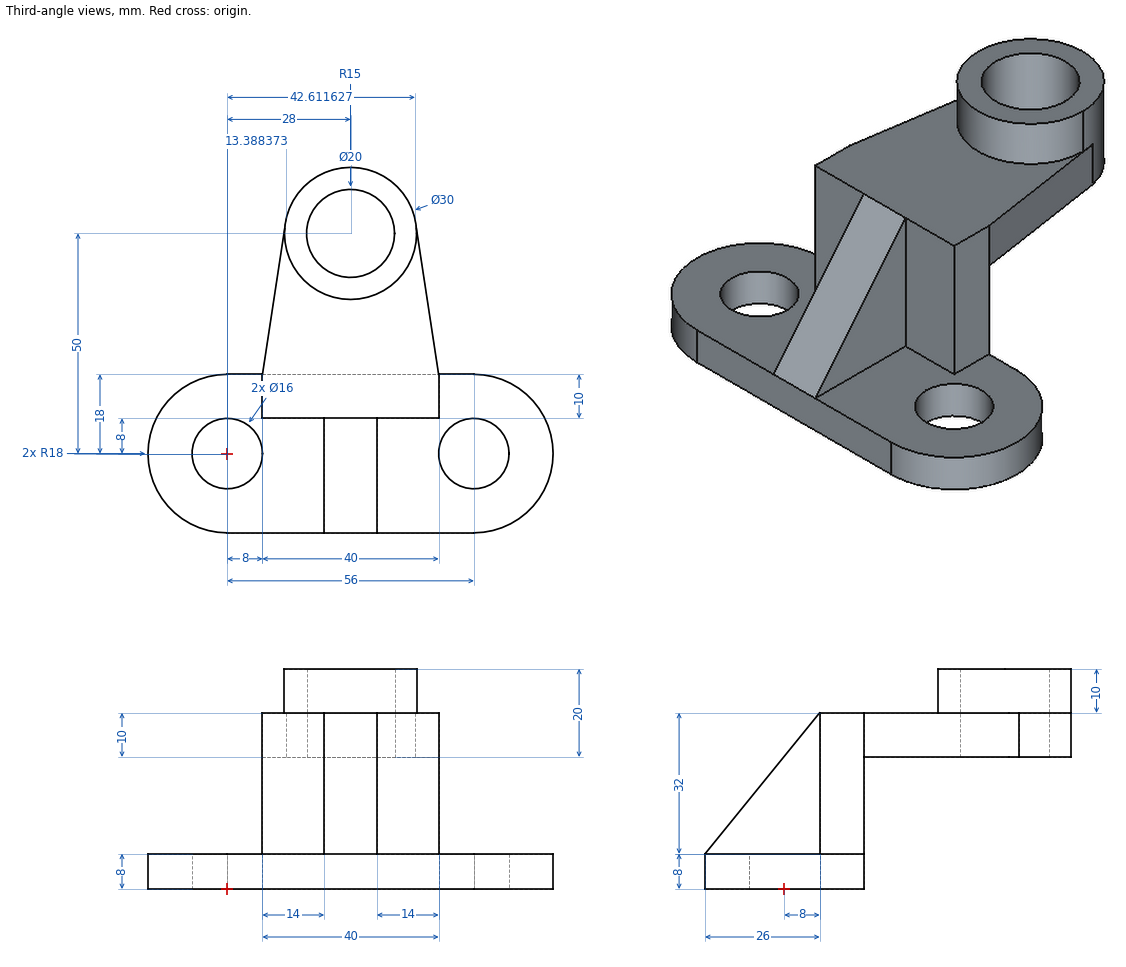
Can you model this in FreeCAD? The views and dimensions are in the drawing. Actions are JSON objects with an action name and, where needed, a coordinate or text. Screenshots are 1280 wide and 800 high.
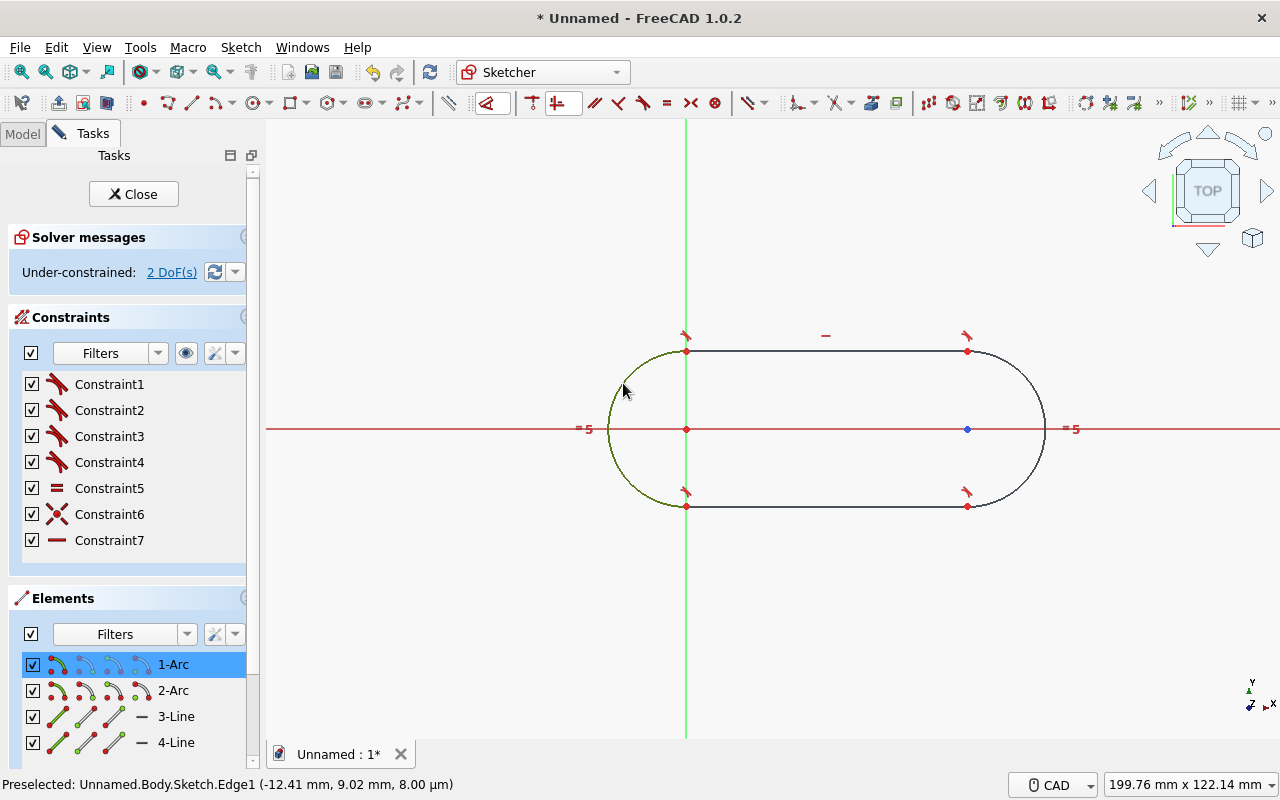
{"action": "key", "text": "k r"}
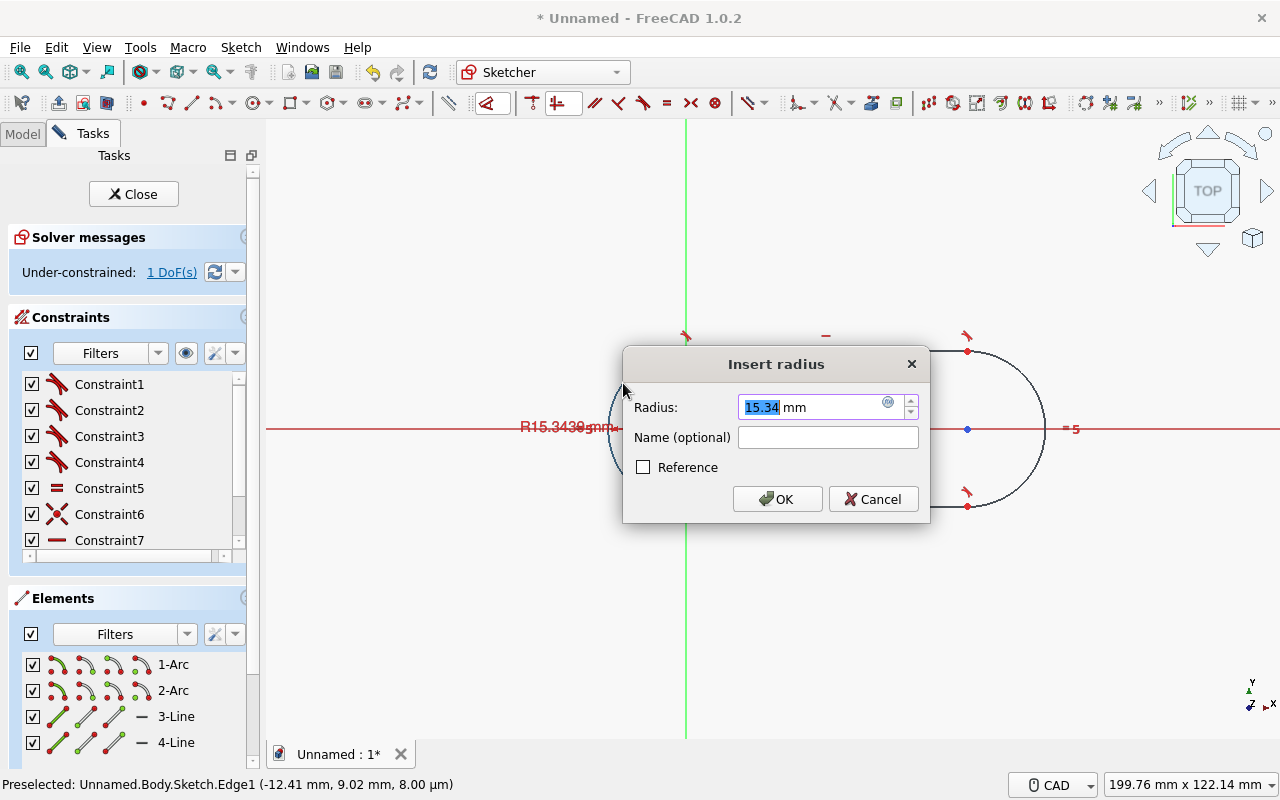
{"action": "type", "text": "18"}
{"action": "key", "text": "Return"}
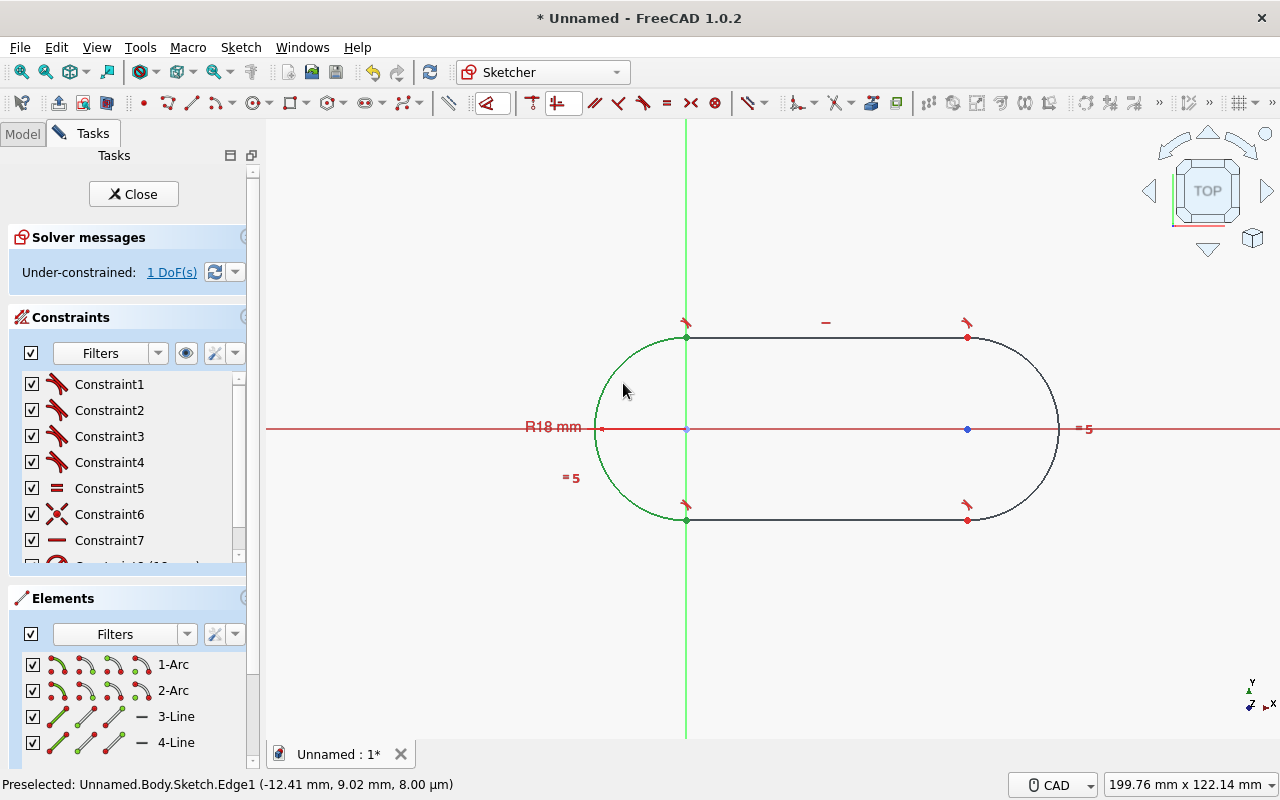
{"action": "left_click", "coordinate": [771, 338]}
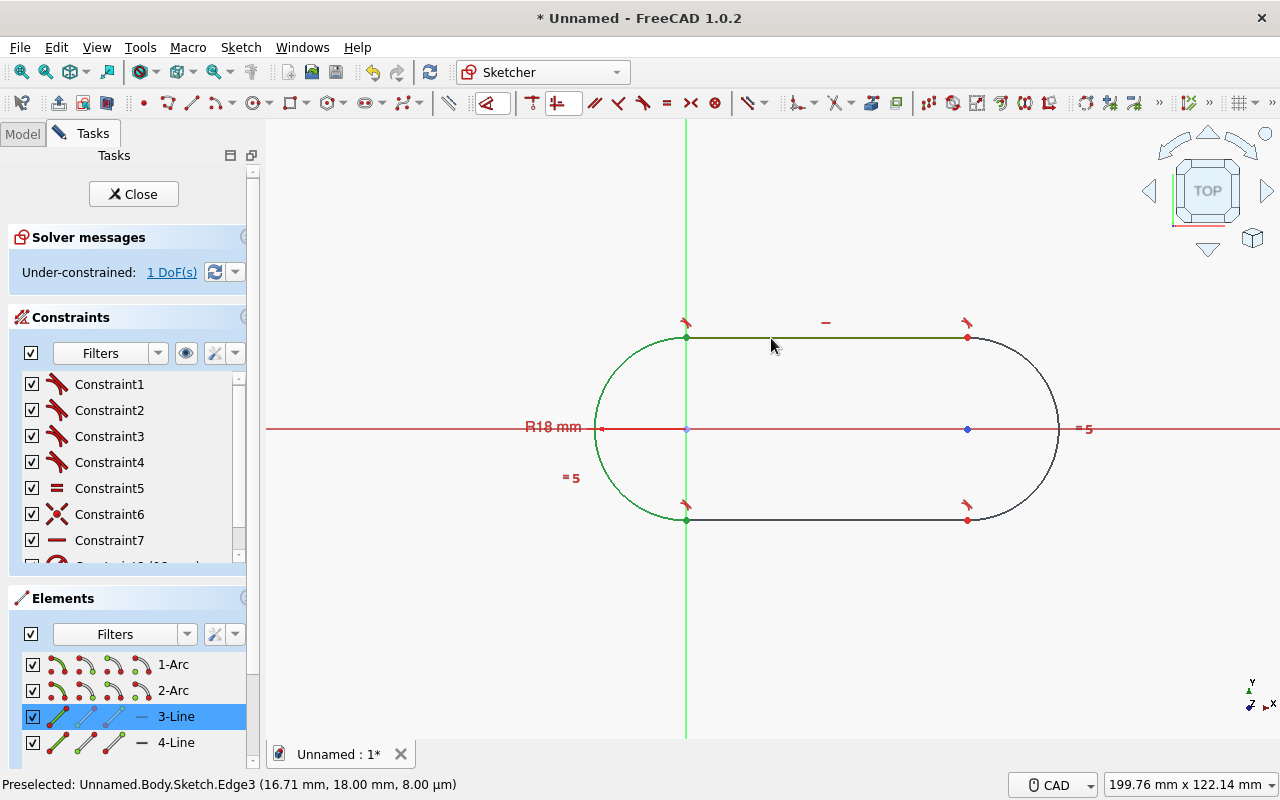
{"action": "left_click", "coordinate": [504, 104]}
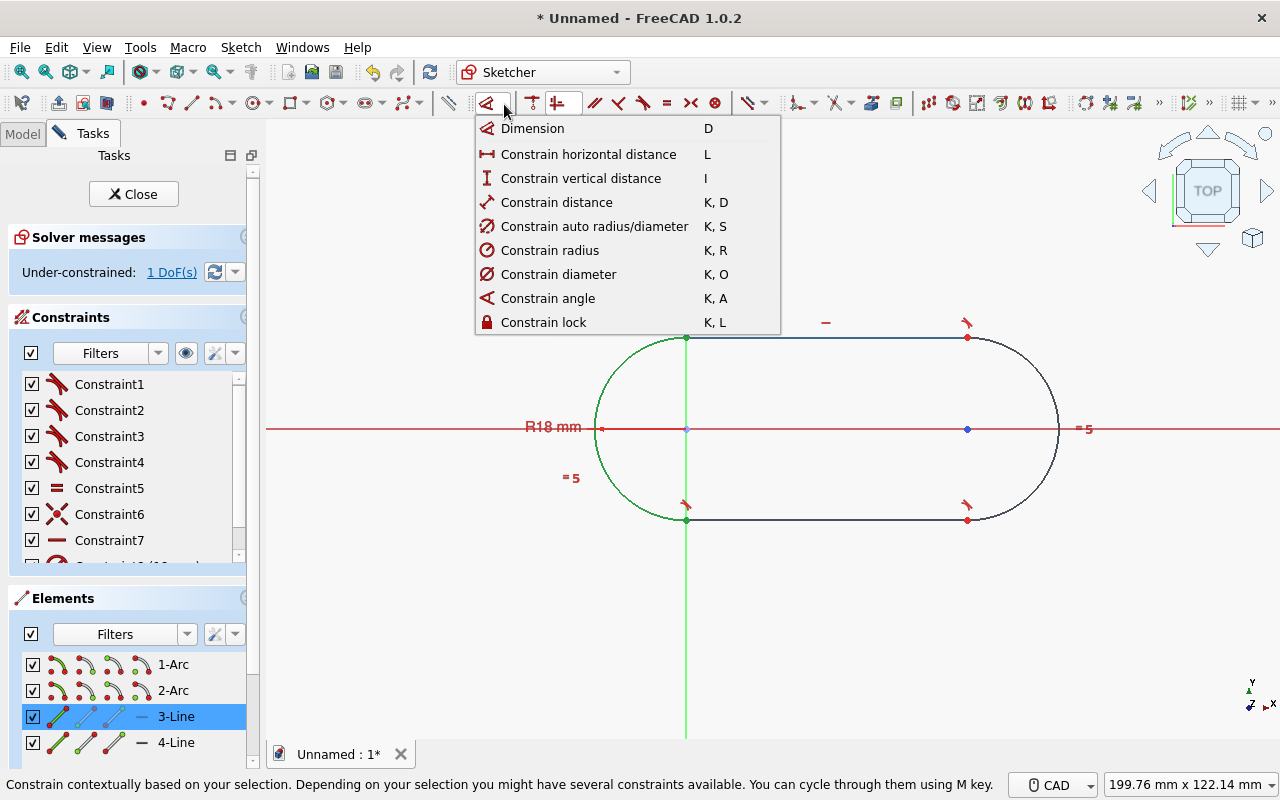
{"action": "left_click", "coordinate": [628, 154]}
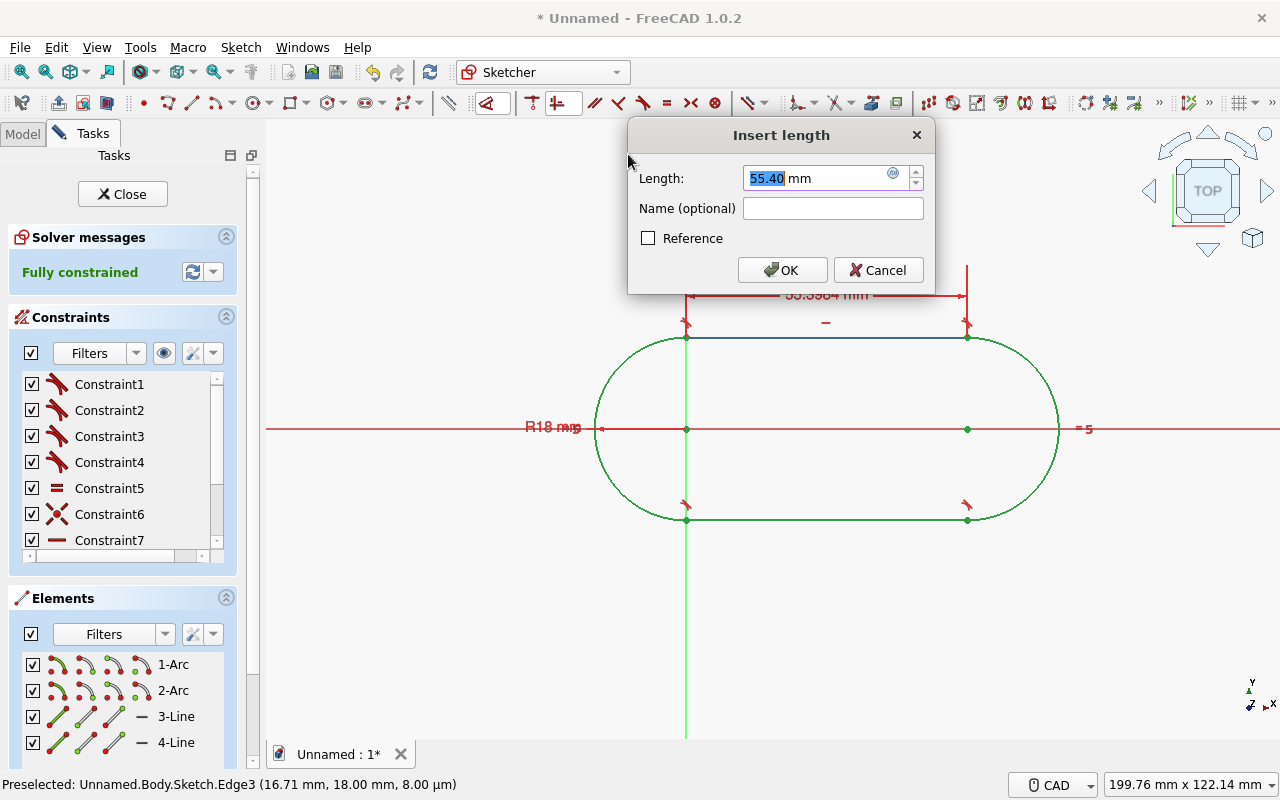
{"action": "type", "text": "56"}
{"action": "key", "text": "Return"}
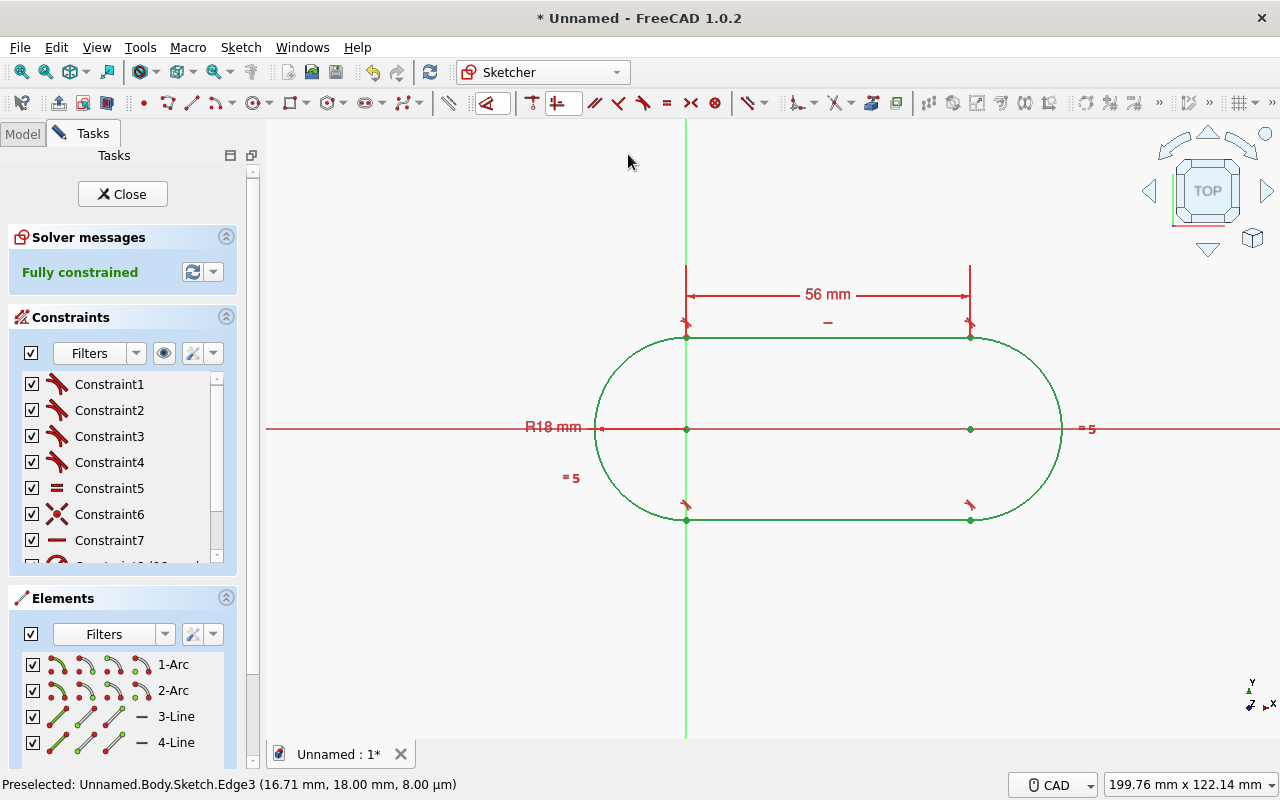
{"action": "left_click", "coordinate": [123, 194]}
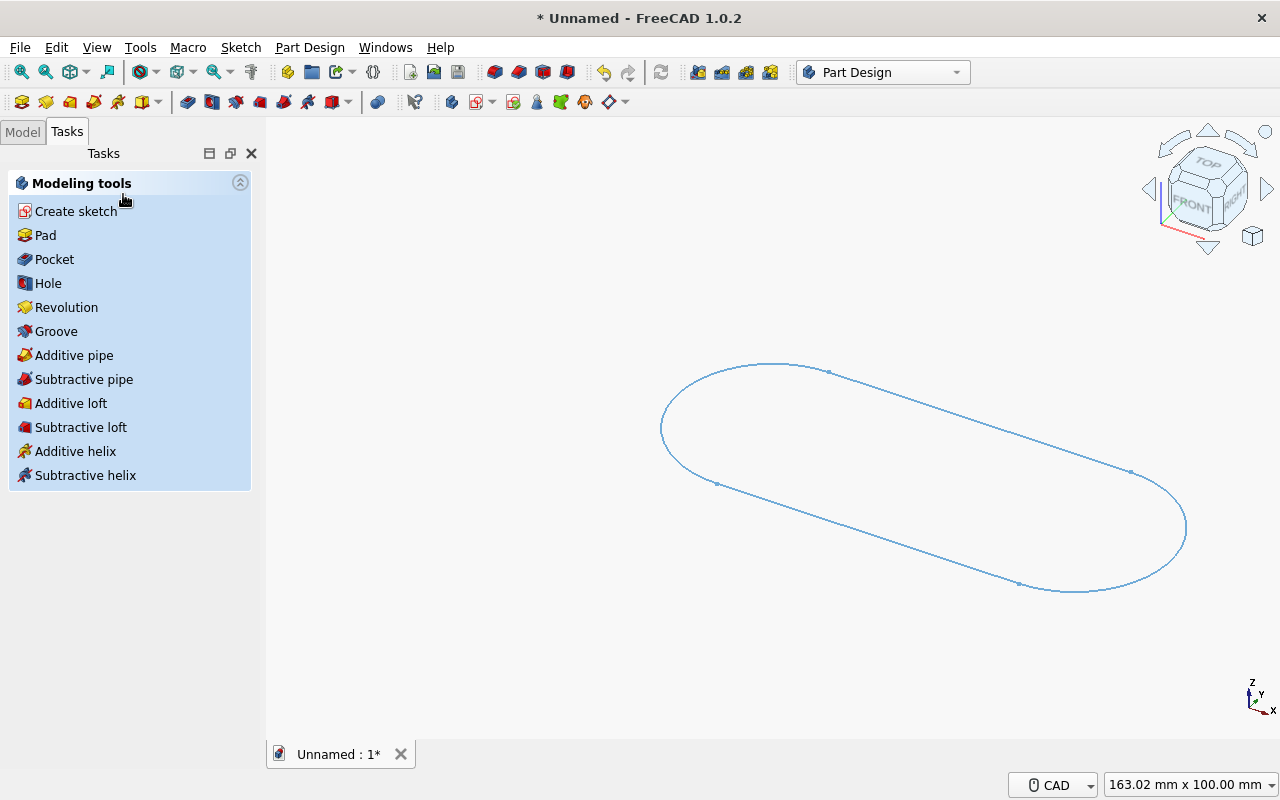
{"action": "left_click", "coordinate": [22, 102]}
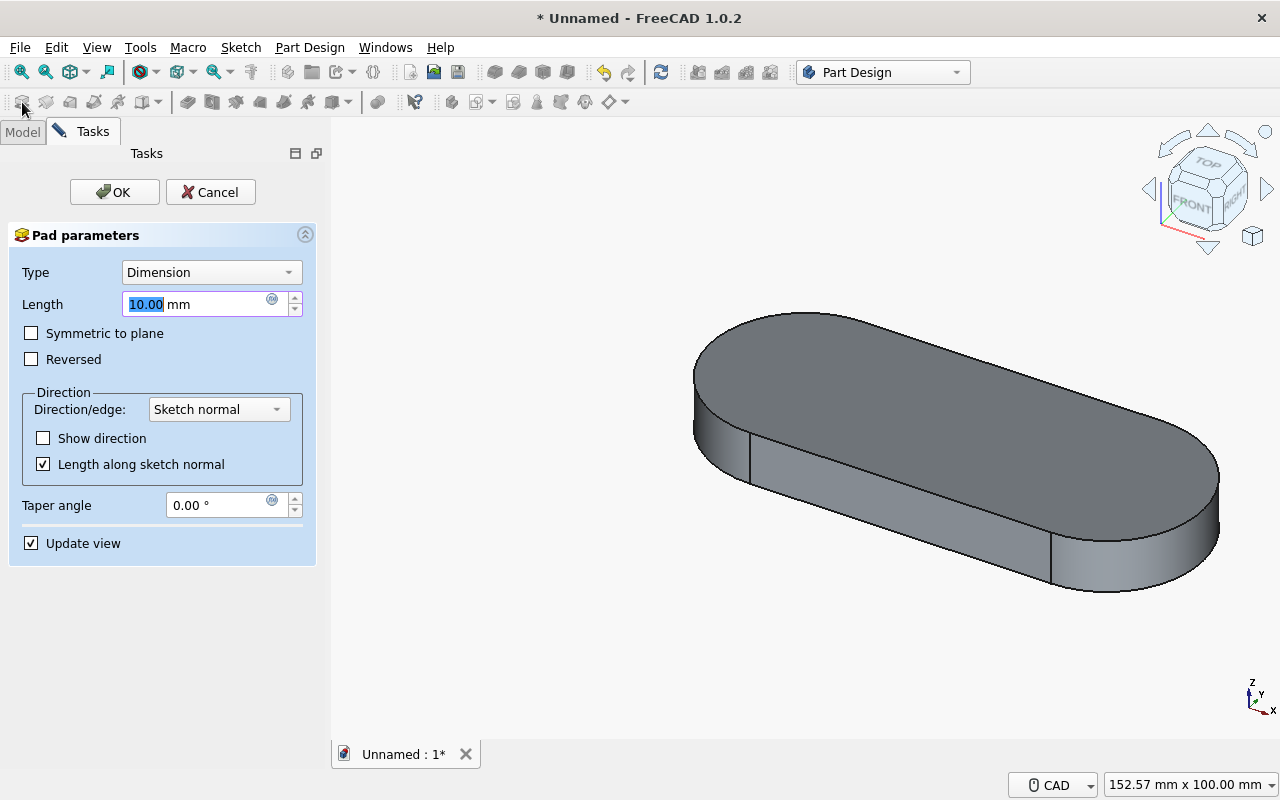
{"action": "type", "text": "8"}
{"action": "key", "text": "Tab"}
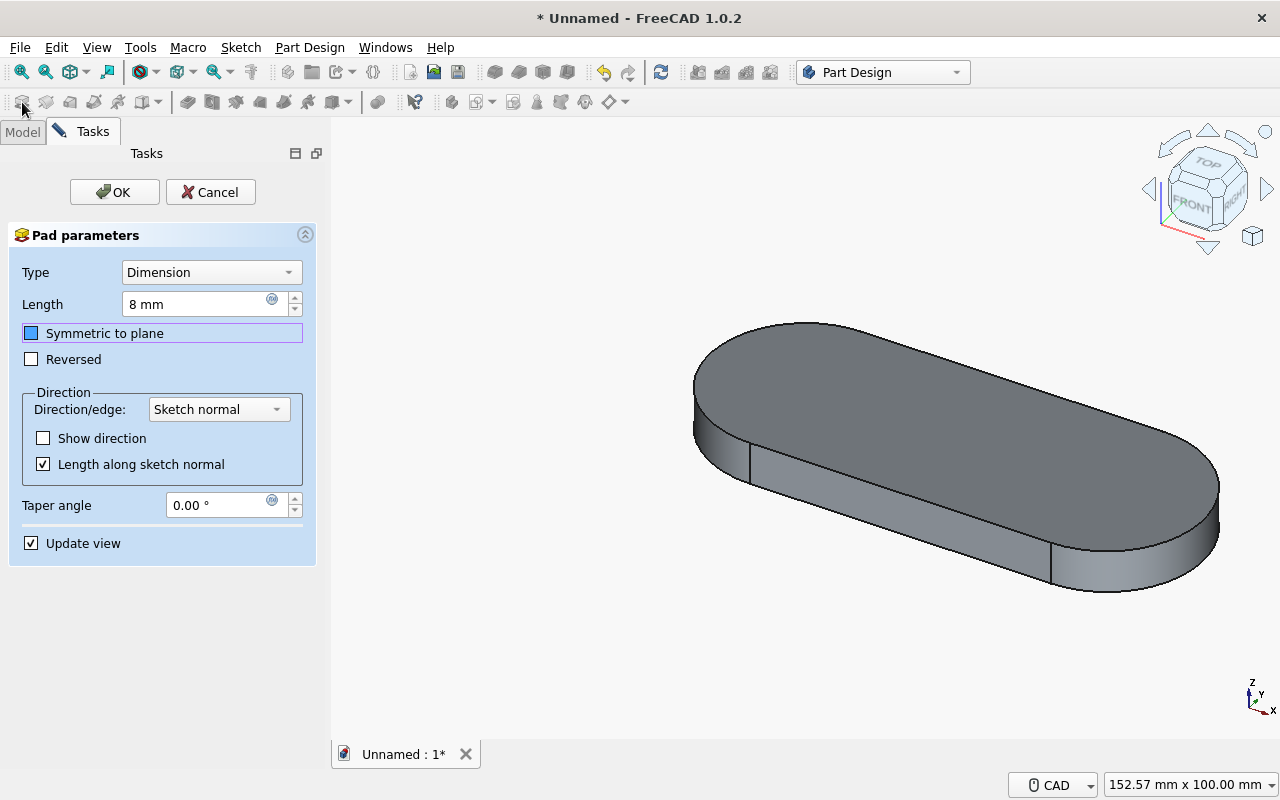
{"action": "left_click", "coordinate": [115, 192]}